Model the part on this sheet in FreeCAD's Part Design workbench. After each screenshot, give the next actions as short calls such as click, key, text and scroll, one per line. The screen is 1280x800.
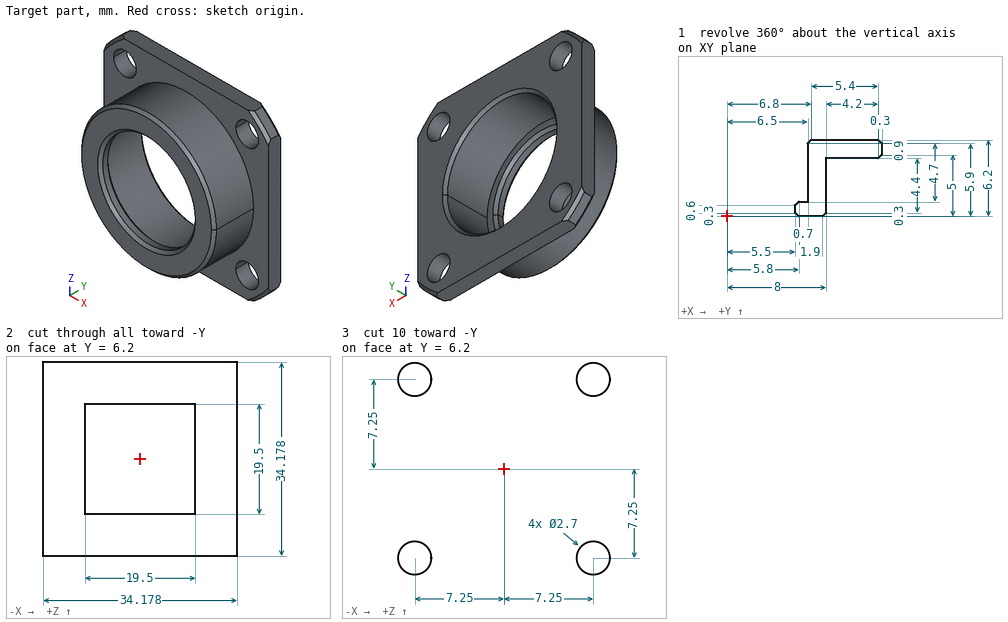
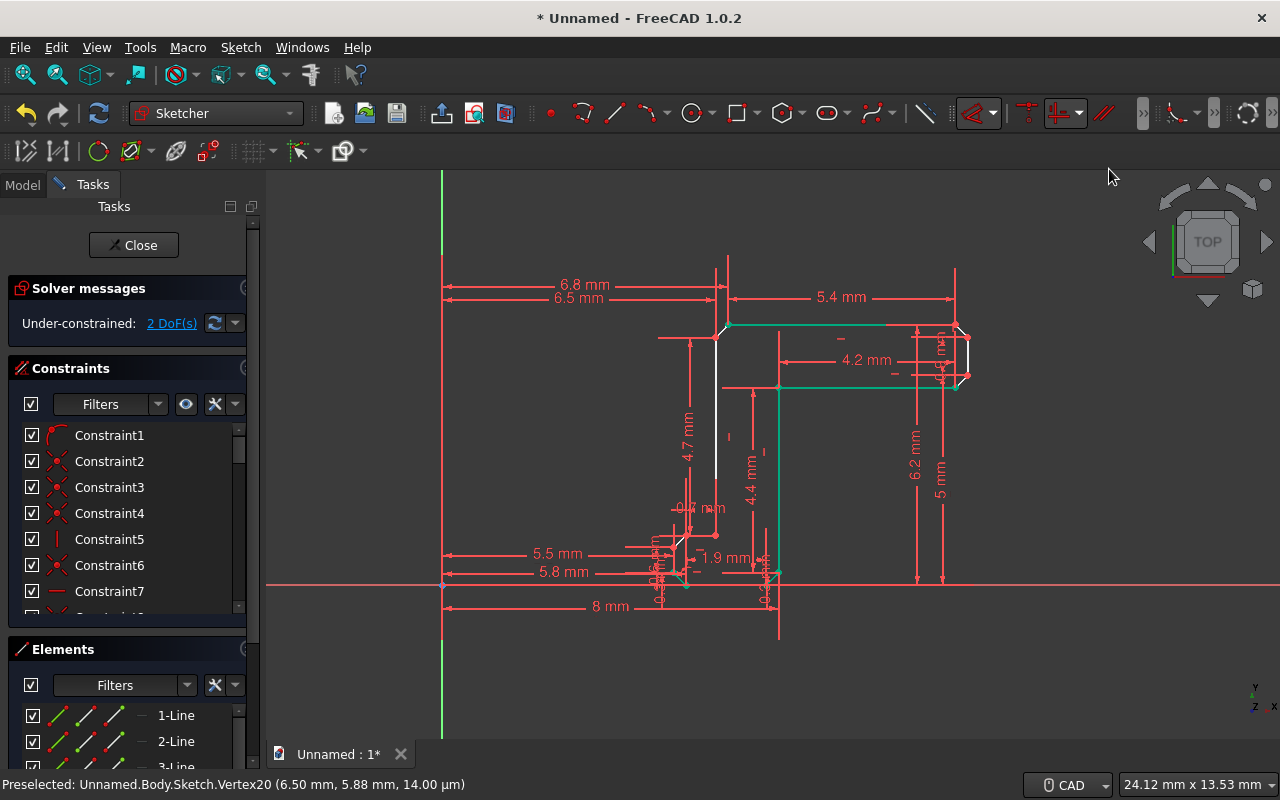
click(716, 338)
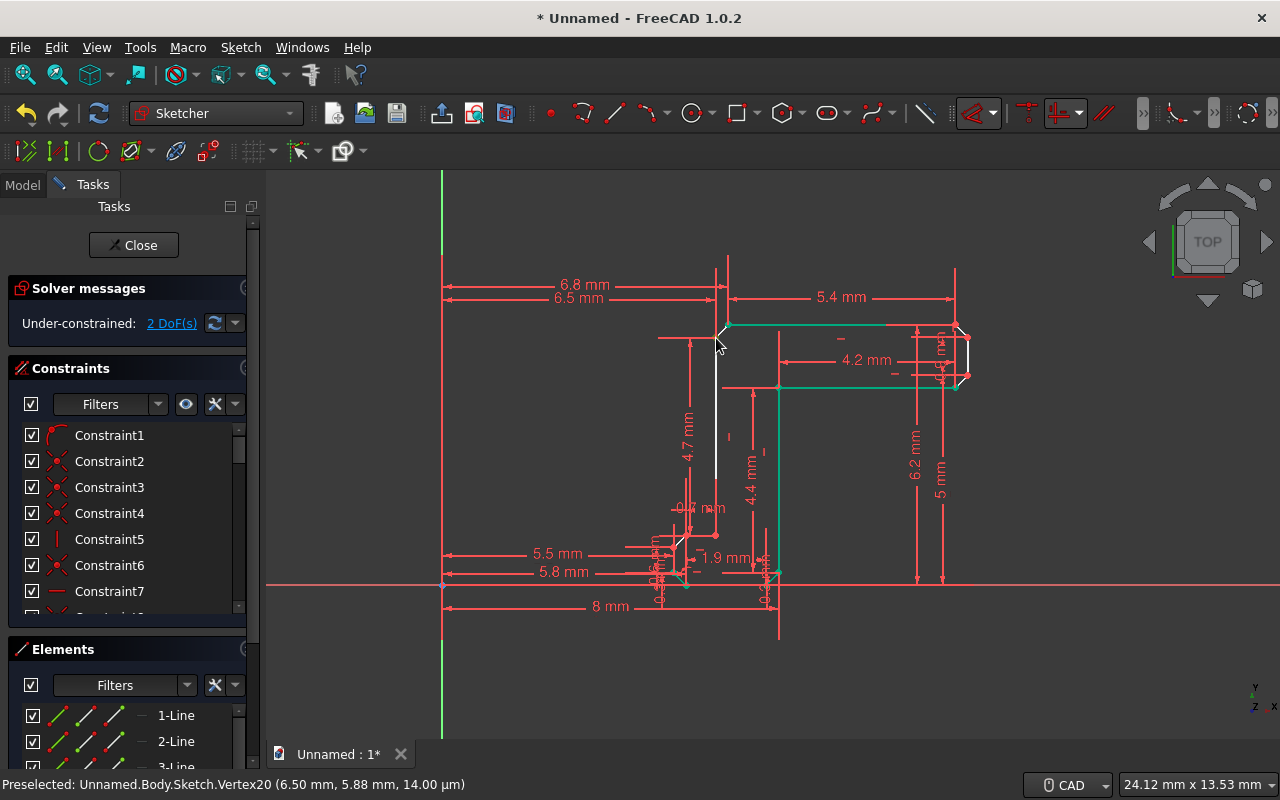
click(996, 114)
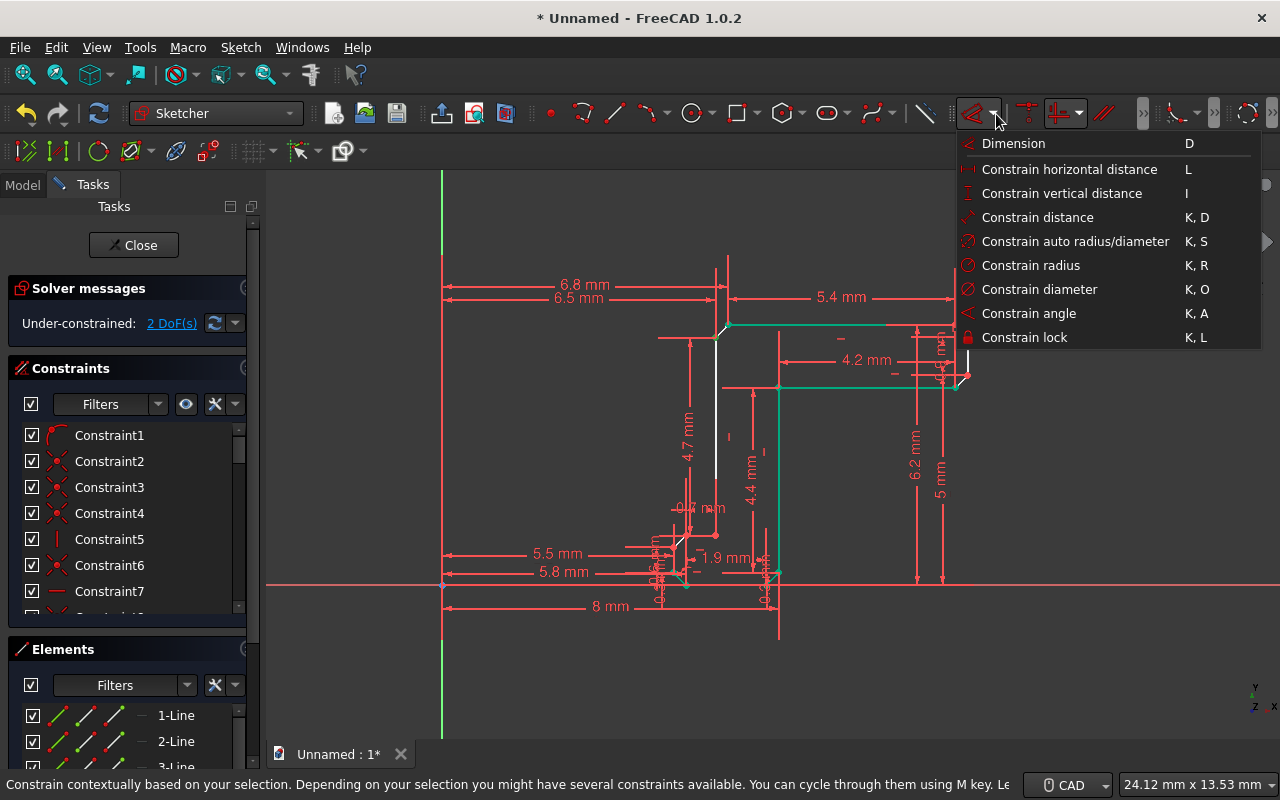
click(1109, 193)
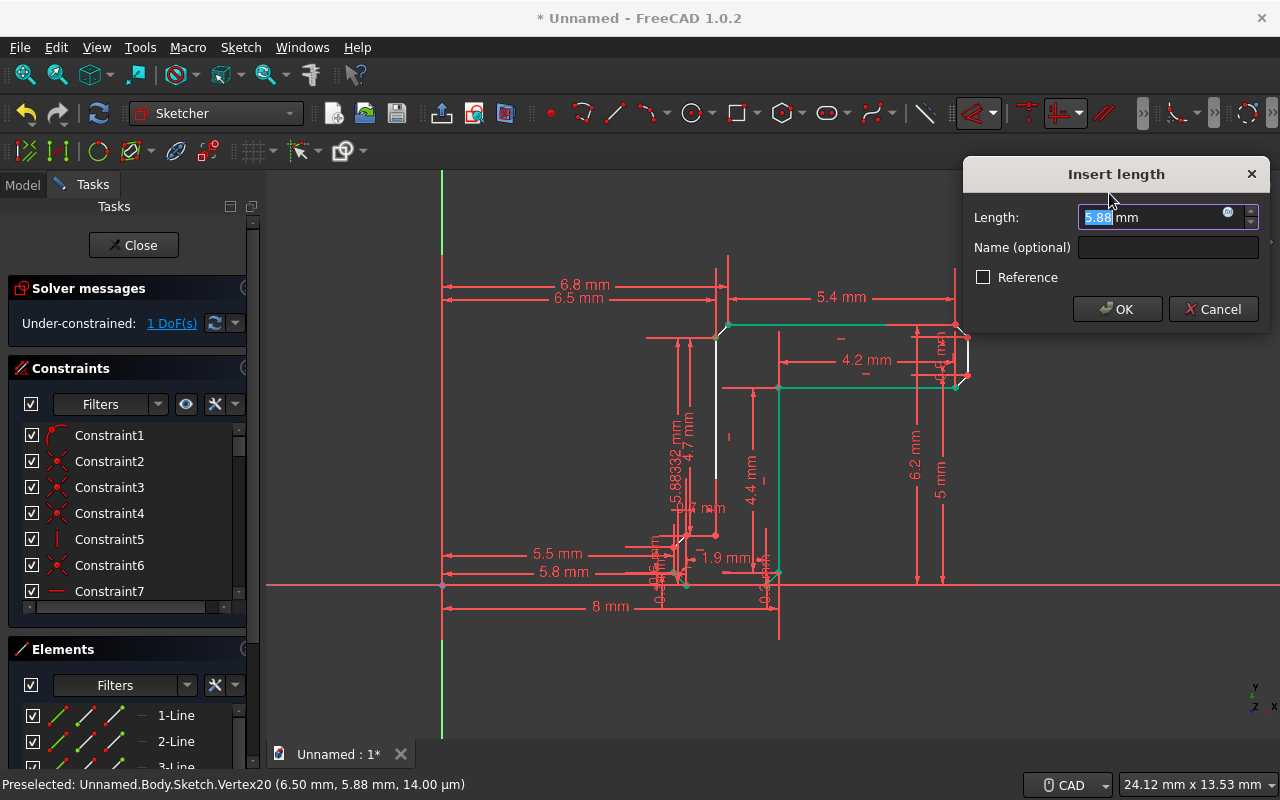
text(5.9)
key(Return)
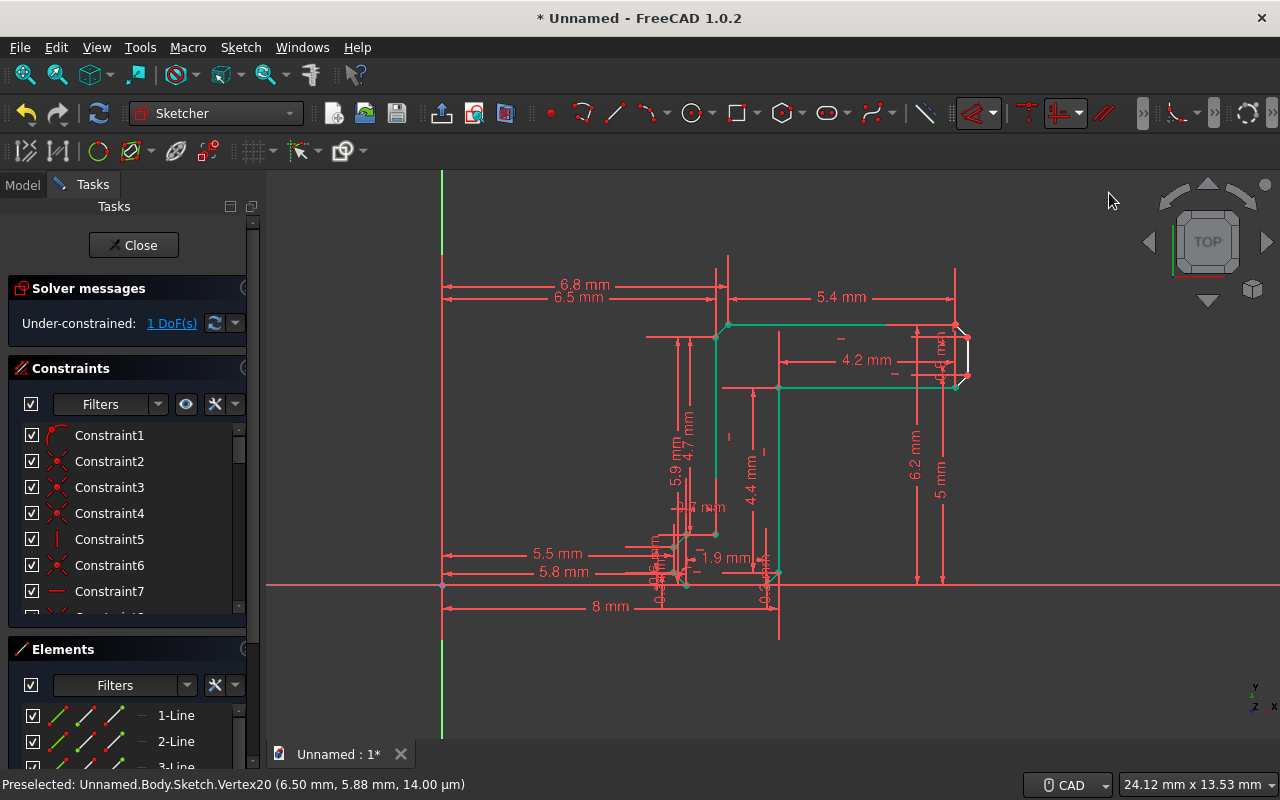
scroll(962, 381, up, 6)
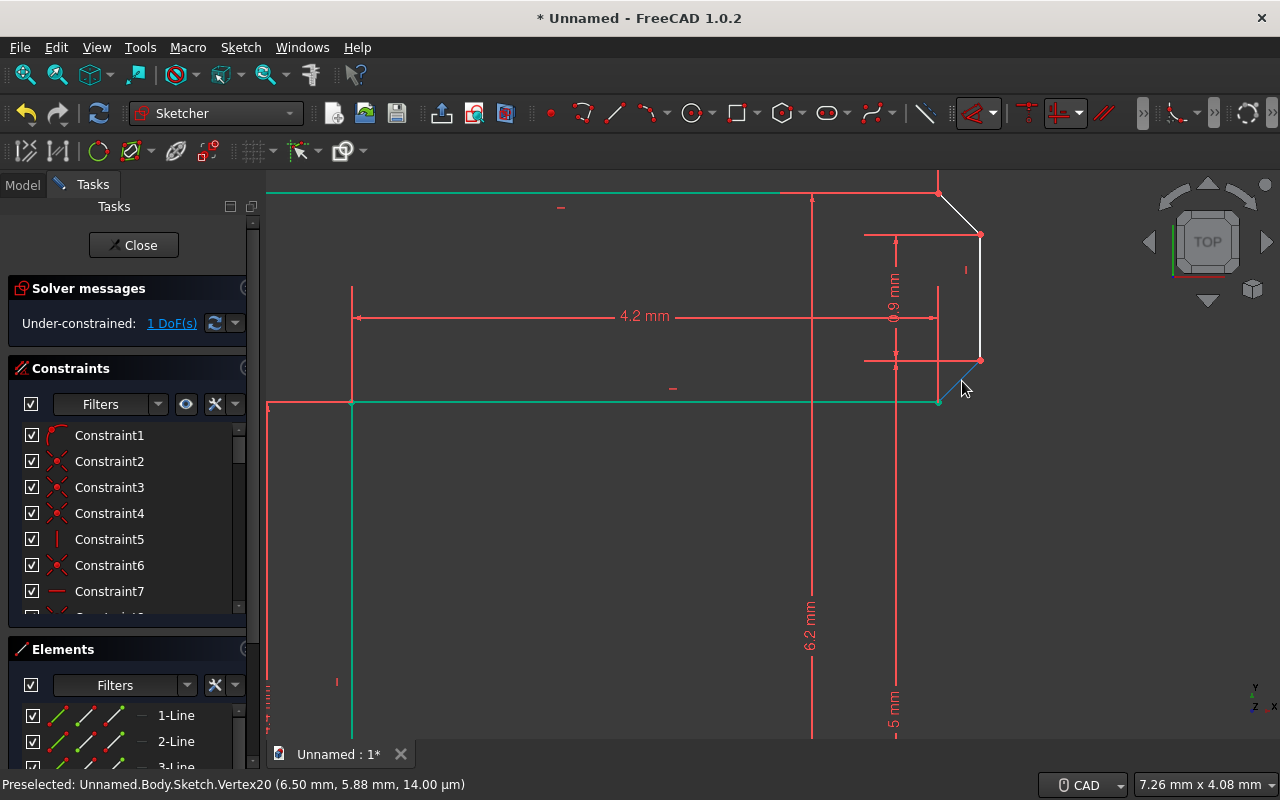
click(959, 381)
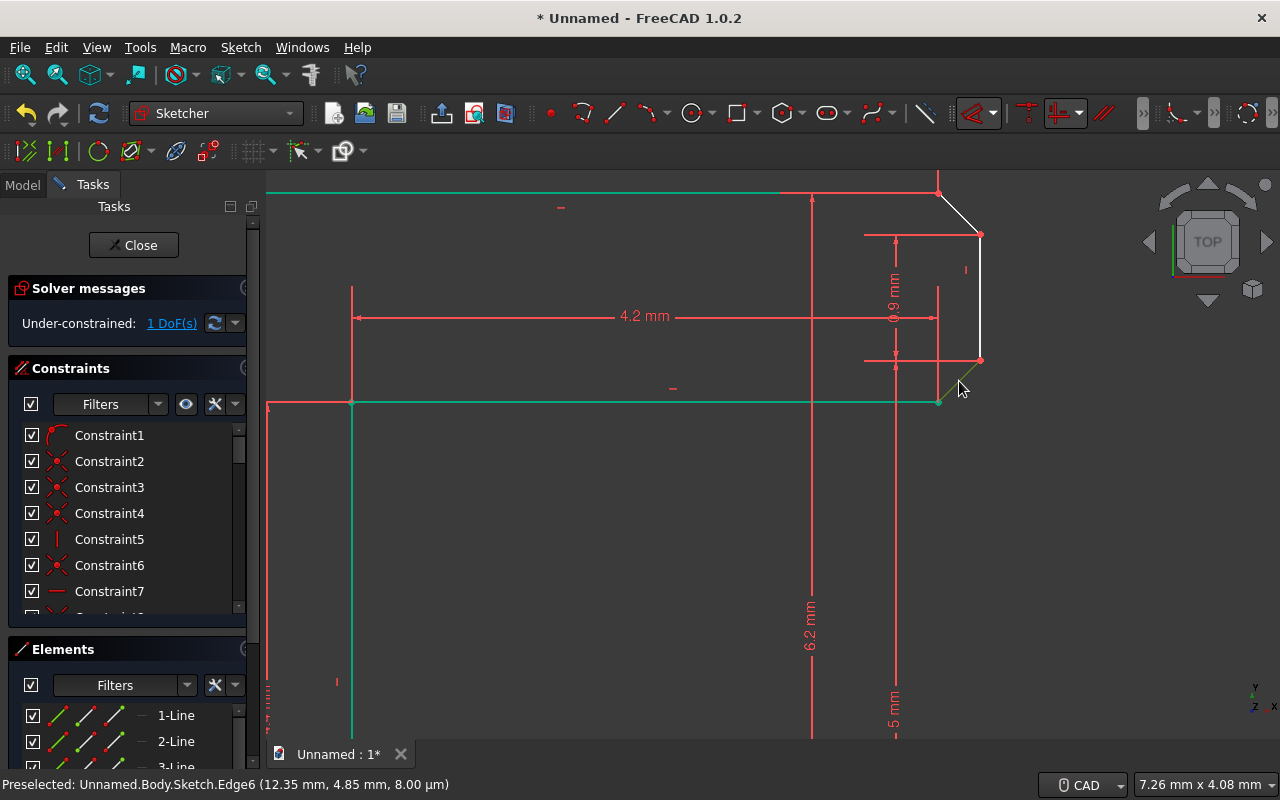
key(l)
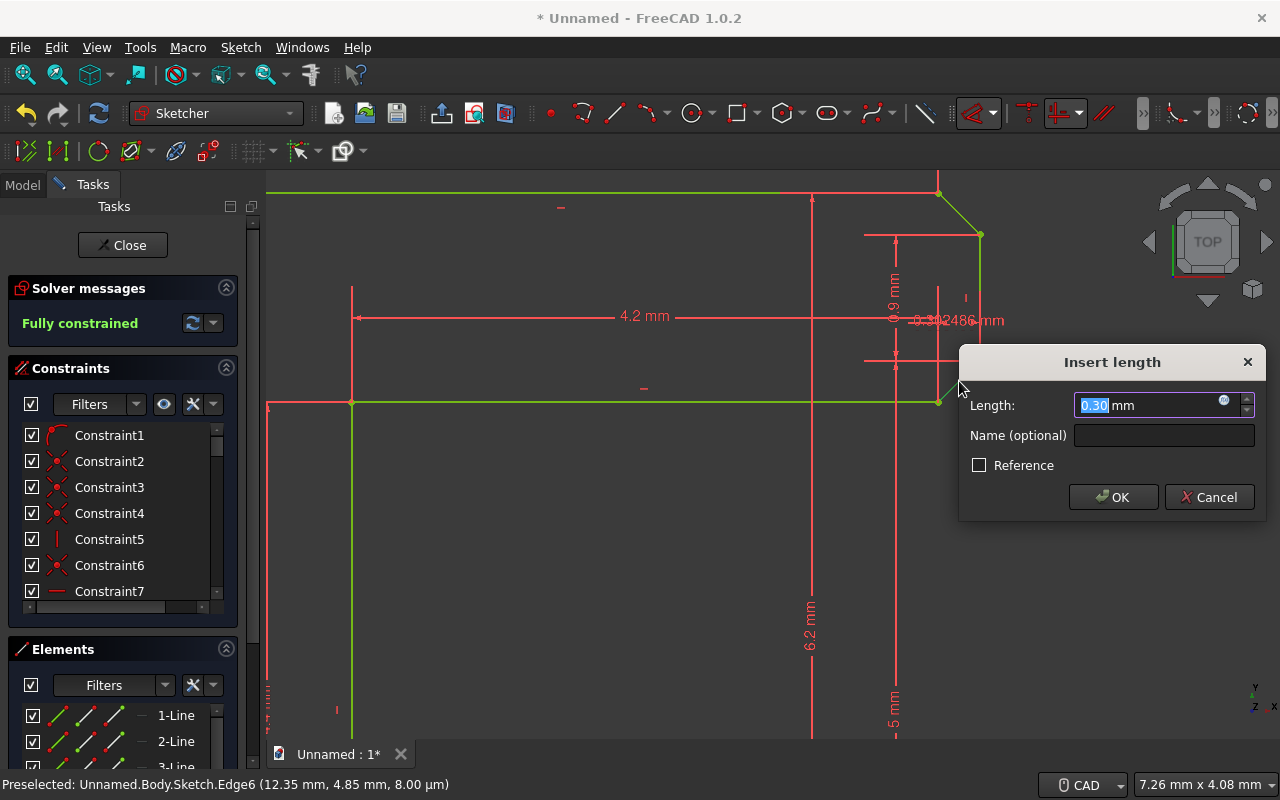
text(0.3)
key(Return)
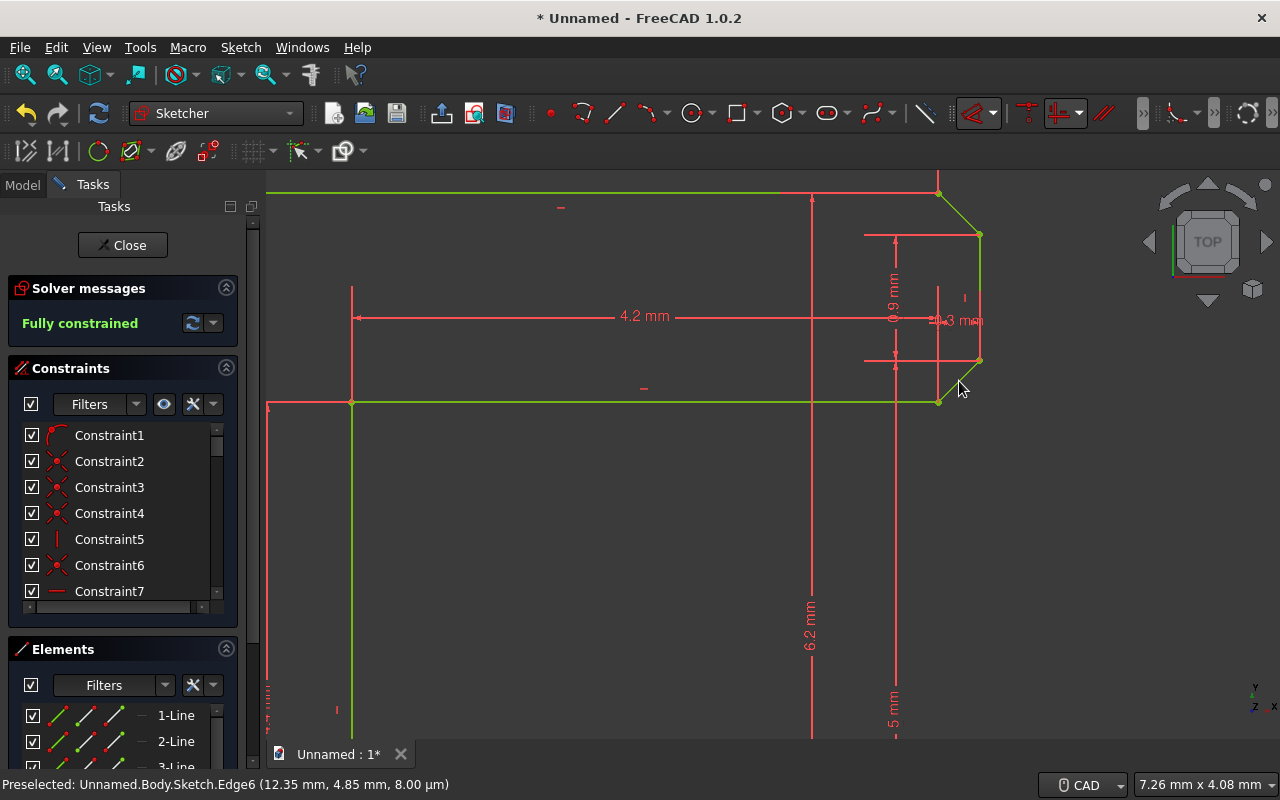
click(123, 245)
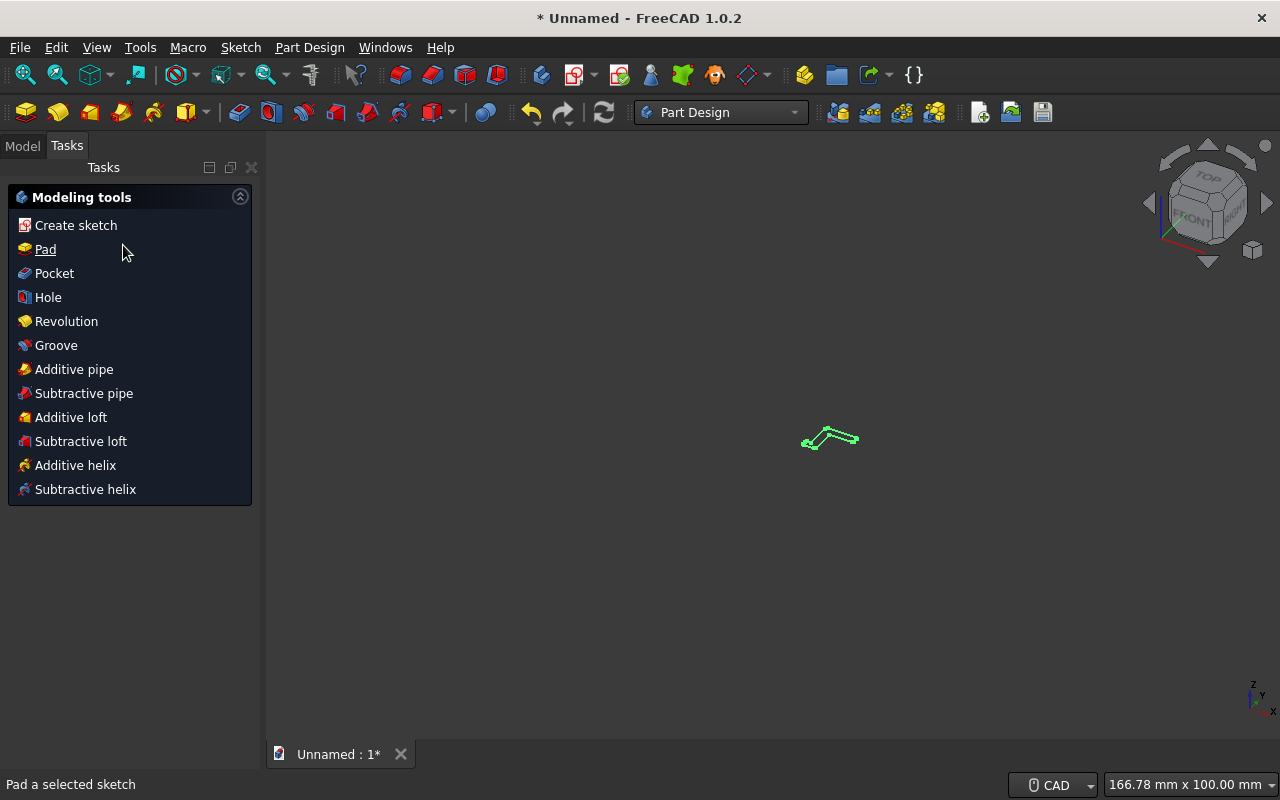
click(58, 112)